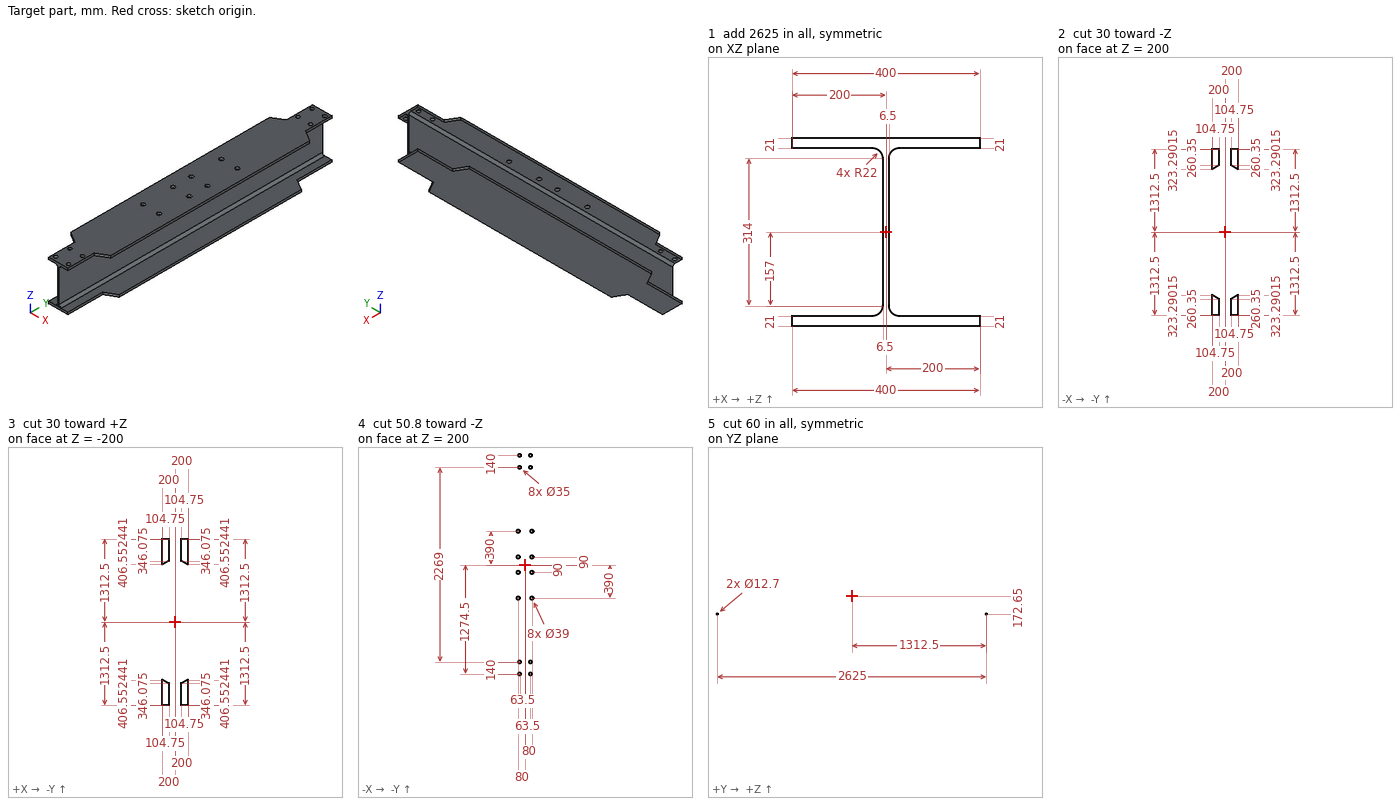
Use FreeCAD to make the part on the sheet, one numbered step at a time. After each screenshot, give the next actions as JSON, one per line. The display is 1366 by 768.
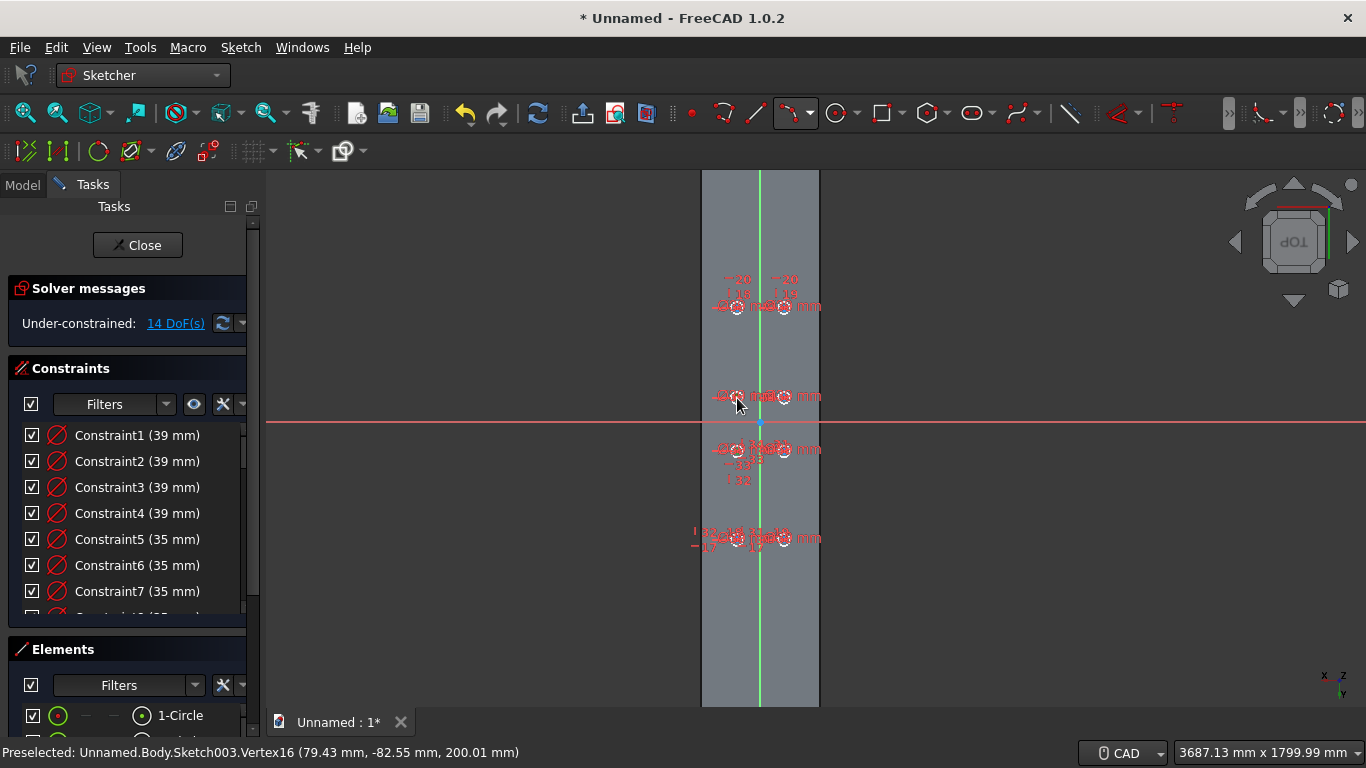
{"action": "key", "text": "v"}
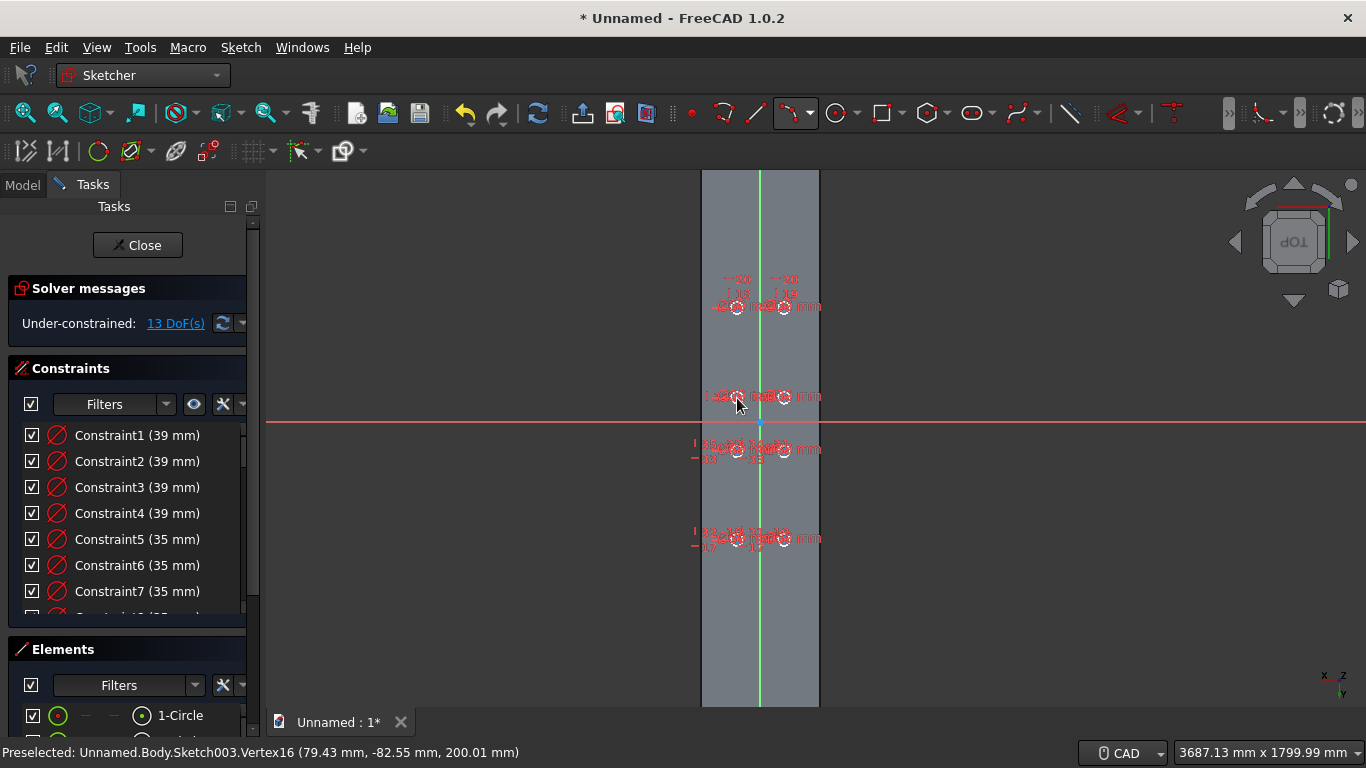
{"action": "left_click", "coordinate": [784, 398]}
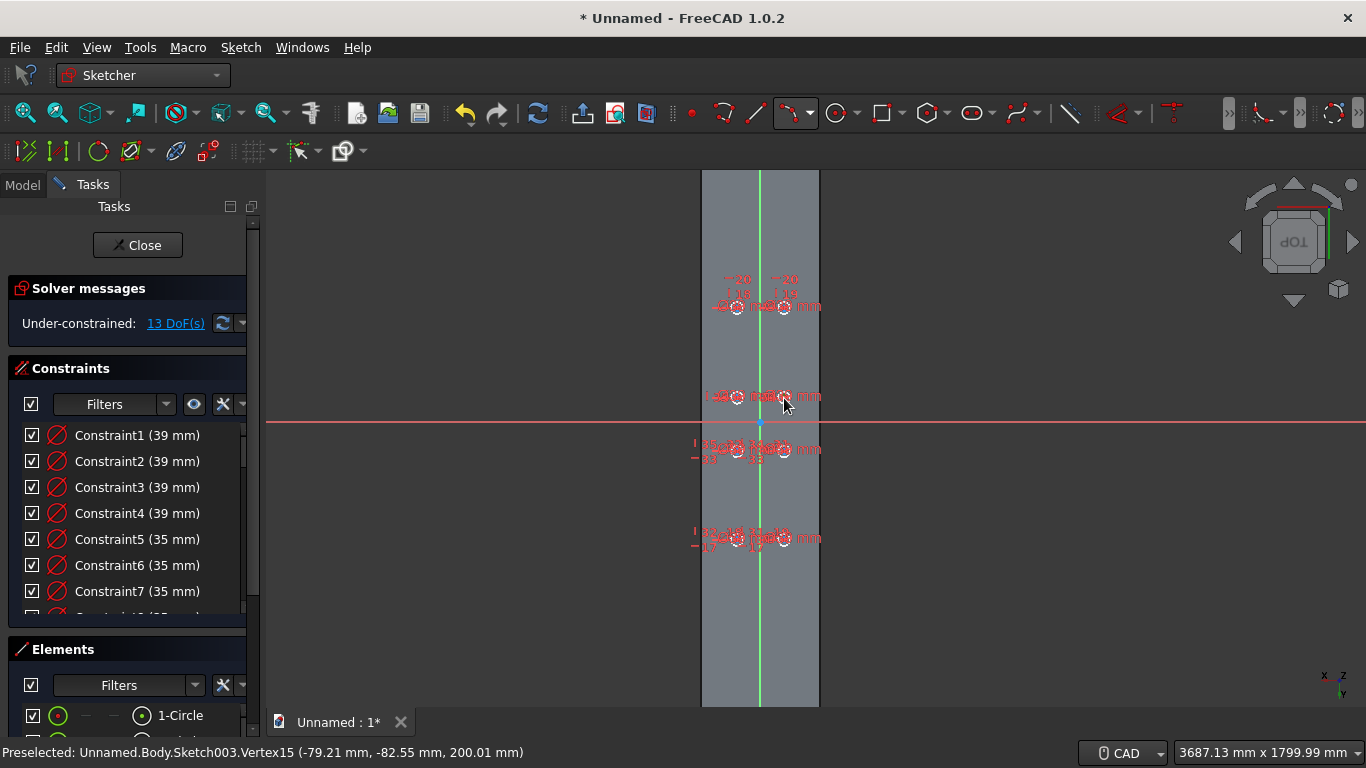
{"action": "left_click", "coordinate": [737, 398]}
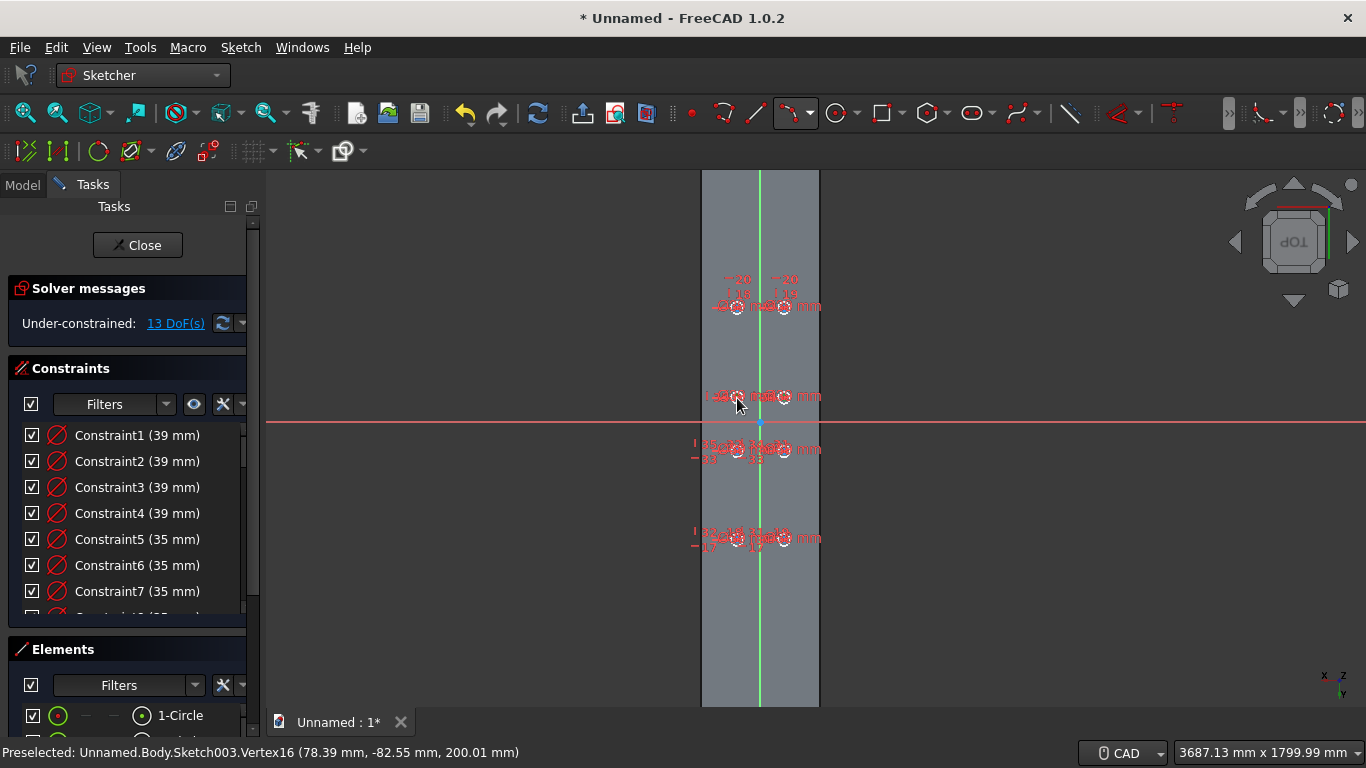
{"action": "key", "text": "h"}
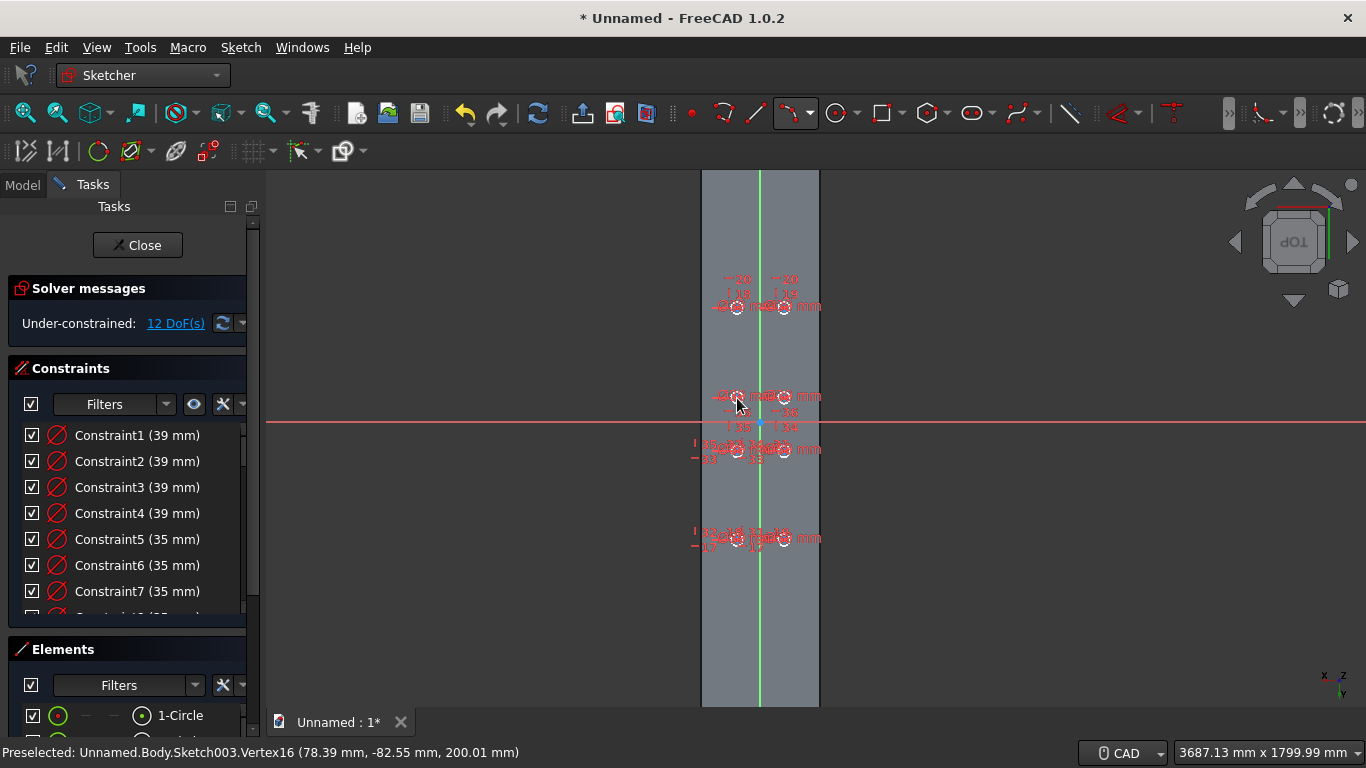
{"action": "left_click", "coordinate": [1118, 114]}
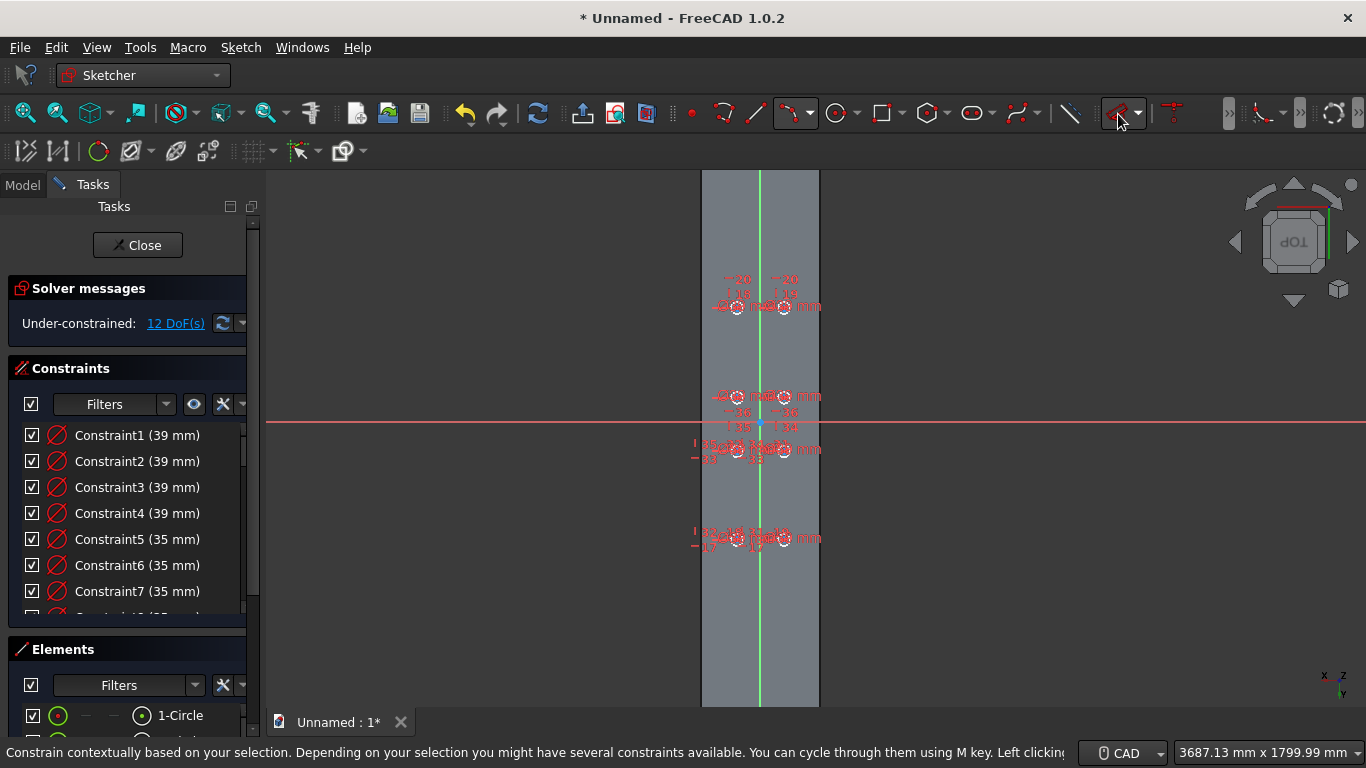
{"action": "scroll", "coordinate": [784, 540], "scroll_direction": "up", "scroll_amount": 3}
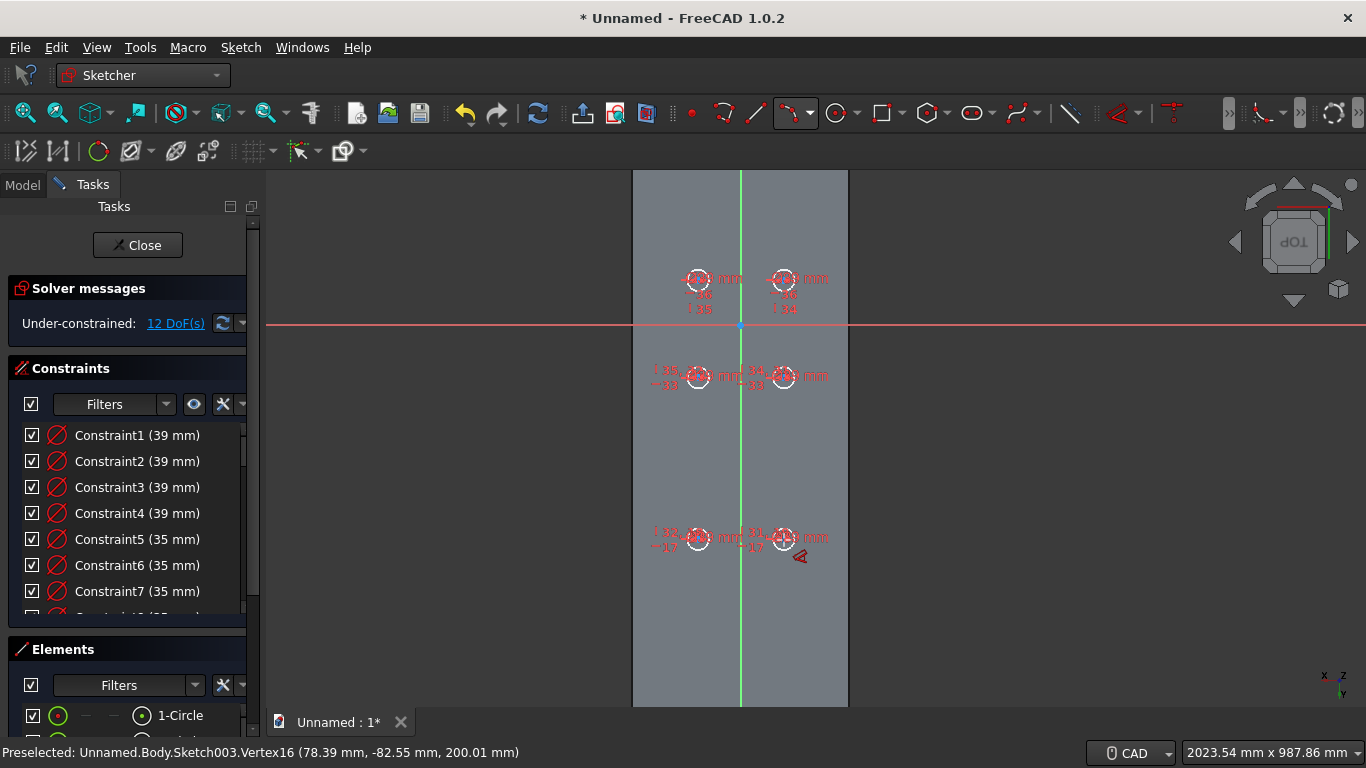
{"action": "left_click", "coordinate": [784, 539]}
{"action": "left_click", "coordinate": [762, 573]}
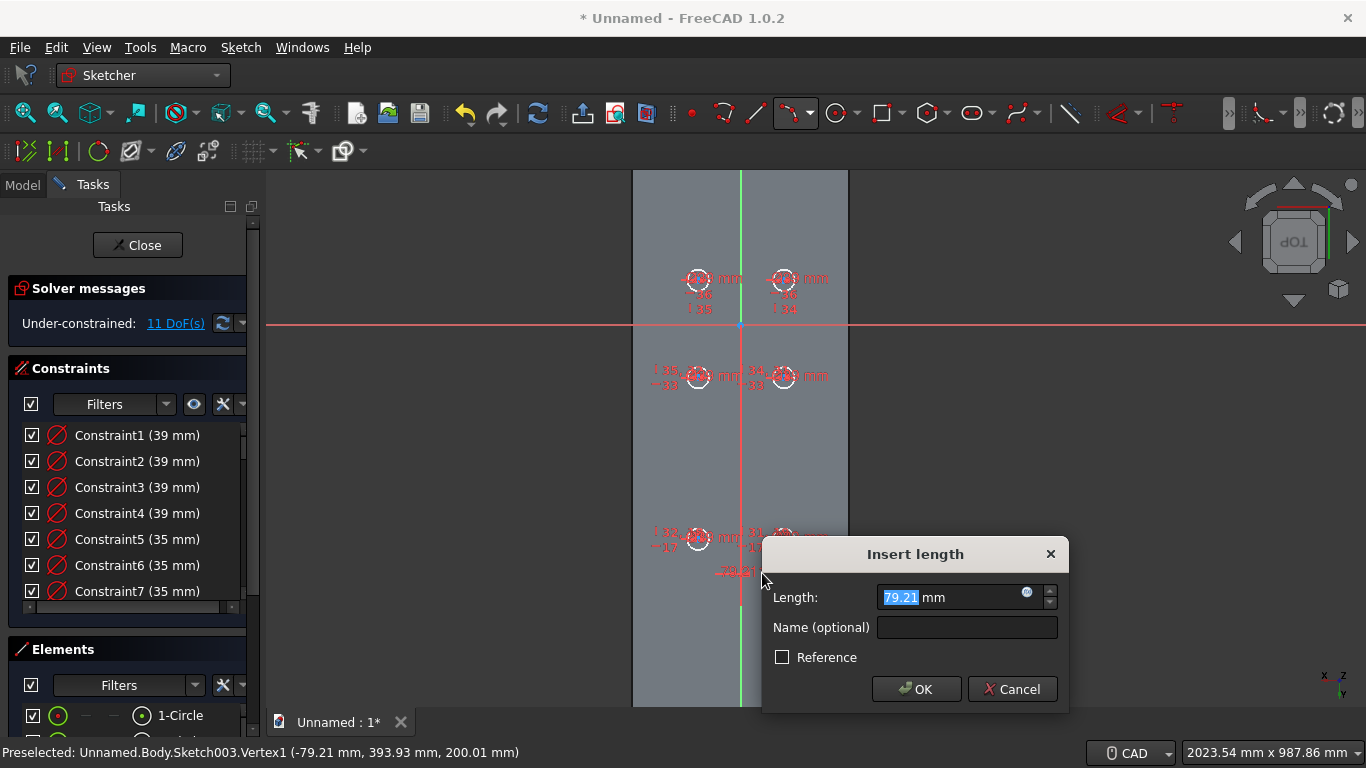
{"action": "type", "text": "80"}
{"action": "key", "text": "Return"}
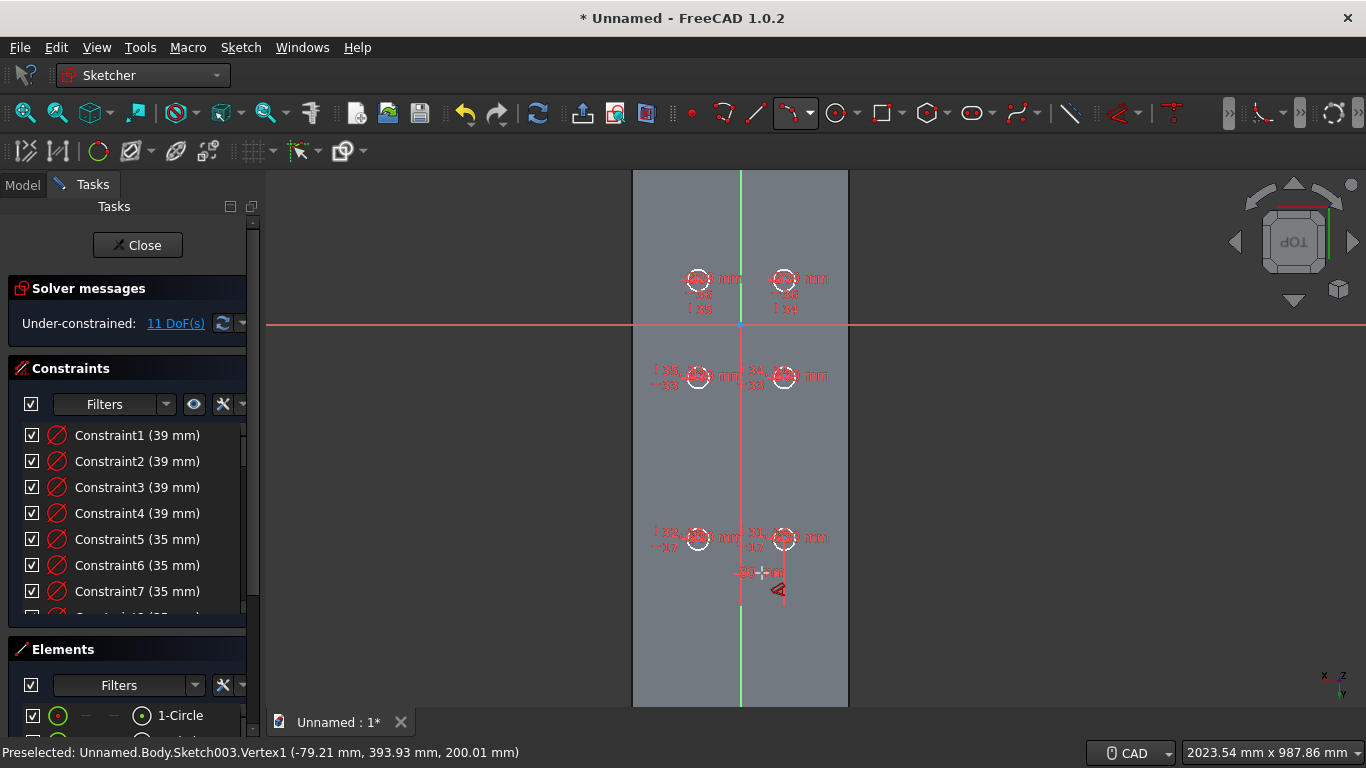
{"action": "left_click", "coordinate": [698, 539]}
{"action": "left_click", "coordinate": [719, 291]}